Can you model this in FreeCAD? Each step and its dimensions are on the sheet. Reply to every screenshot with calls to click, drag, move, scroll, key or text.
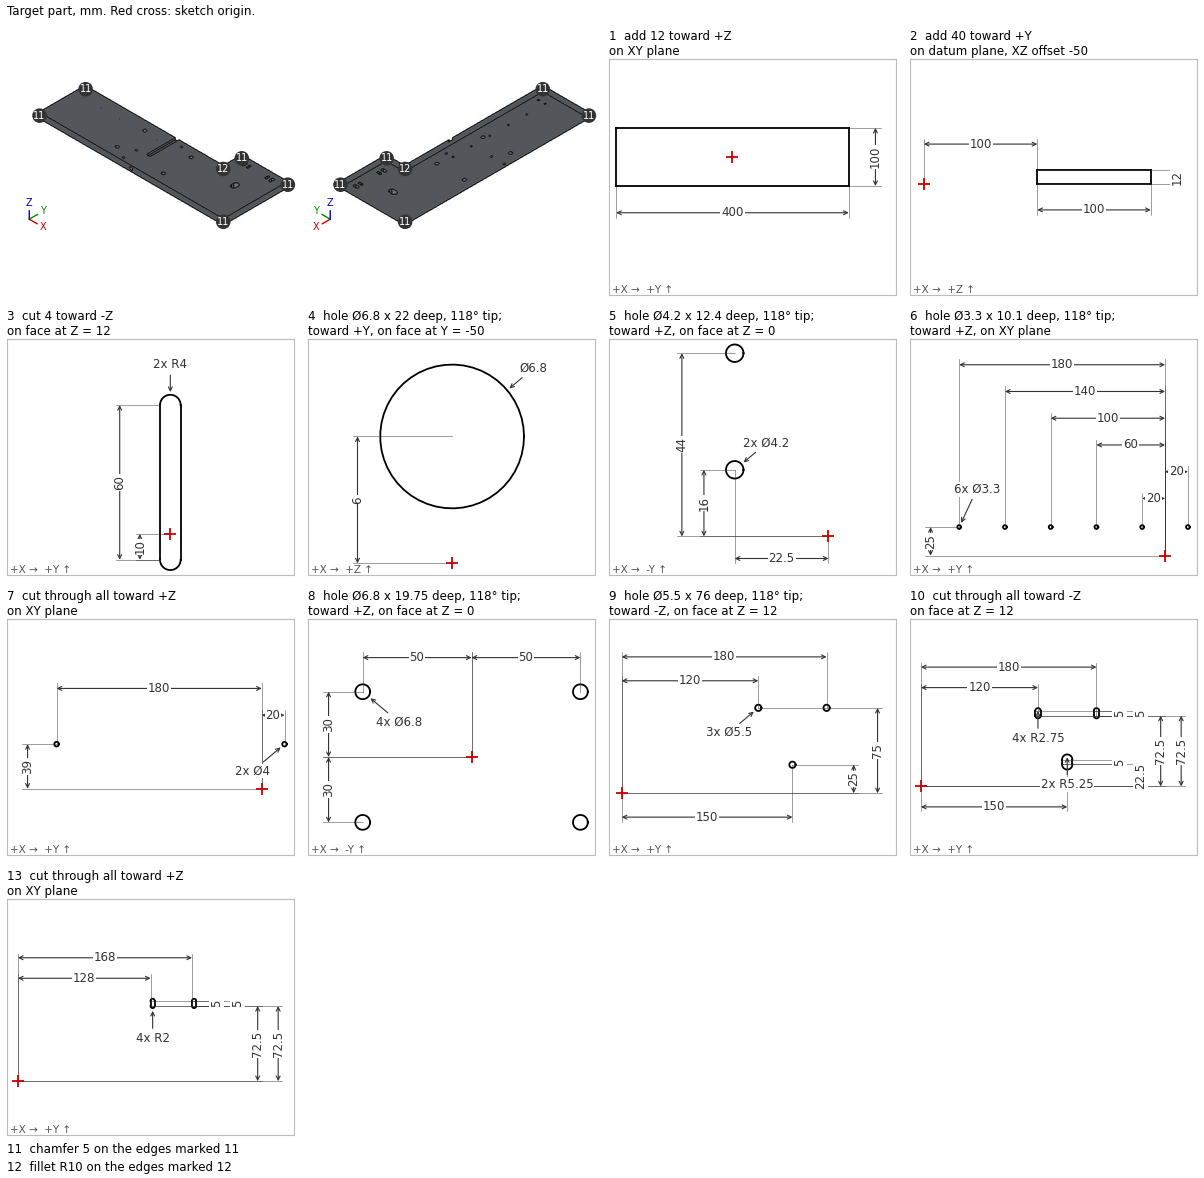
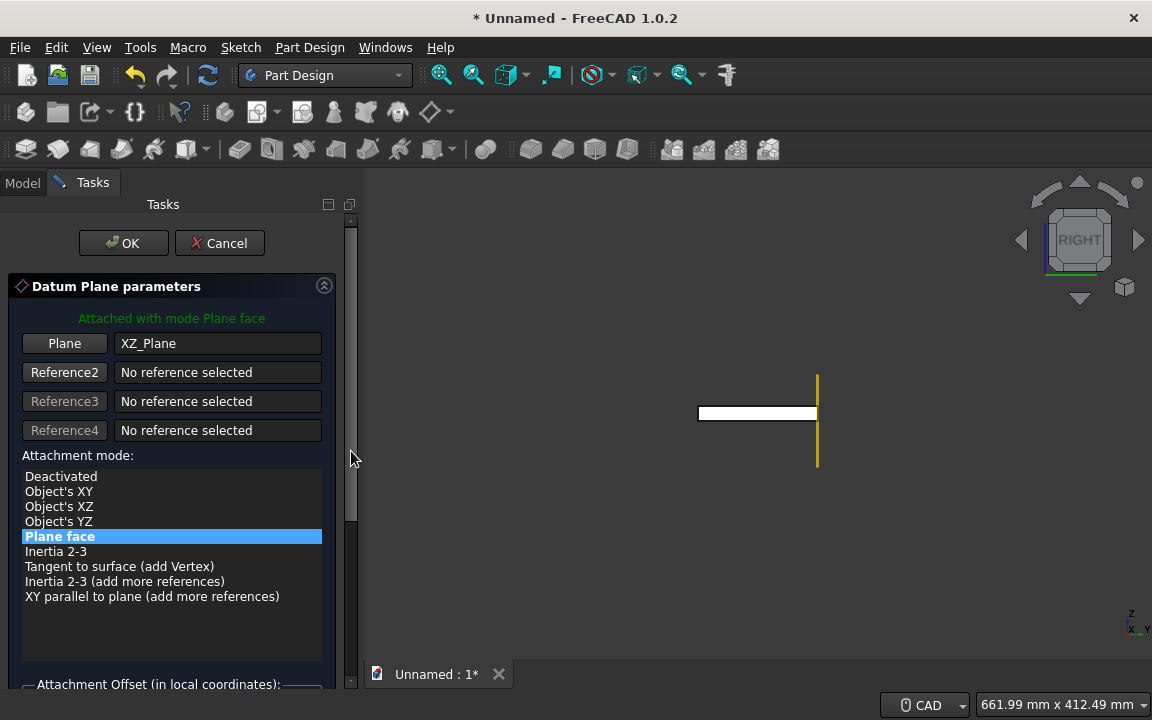
click(124, 243)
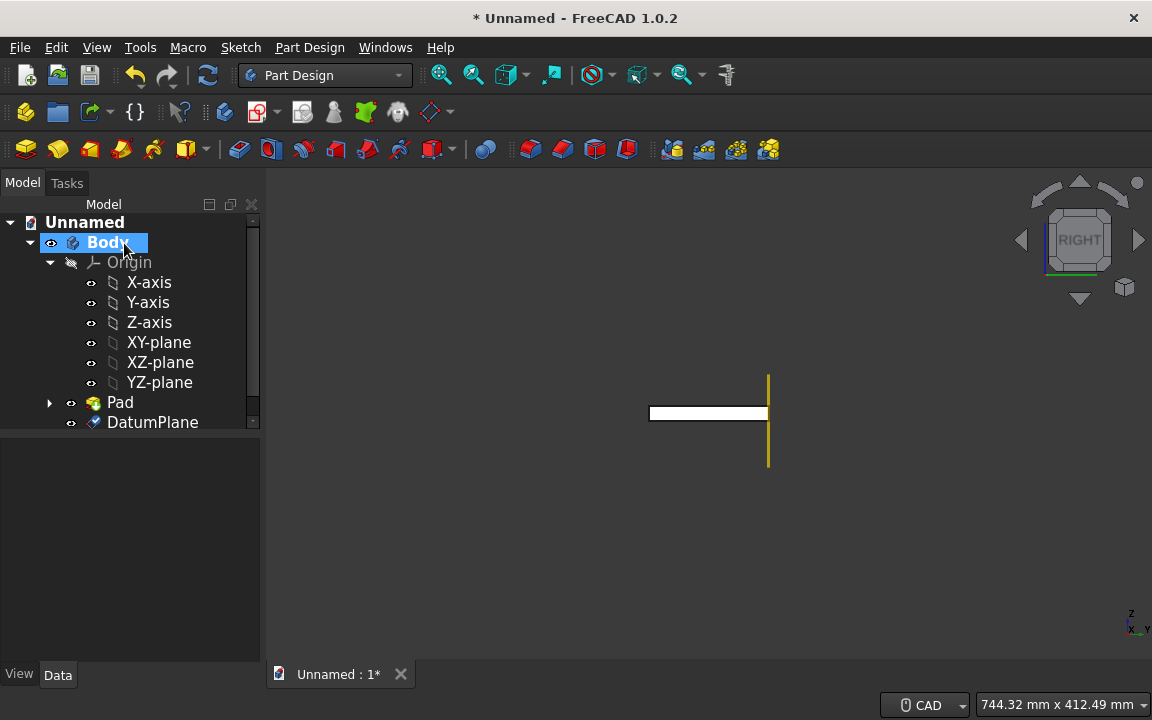
click(116, 423)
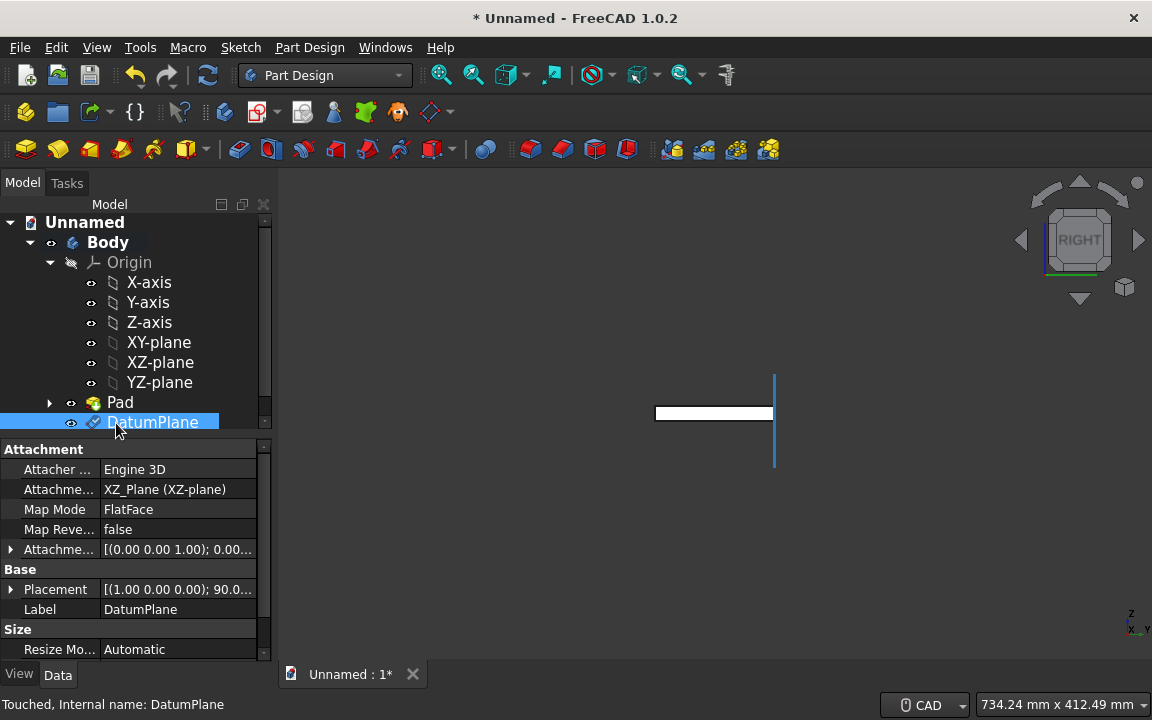
click(258, 112)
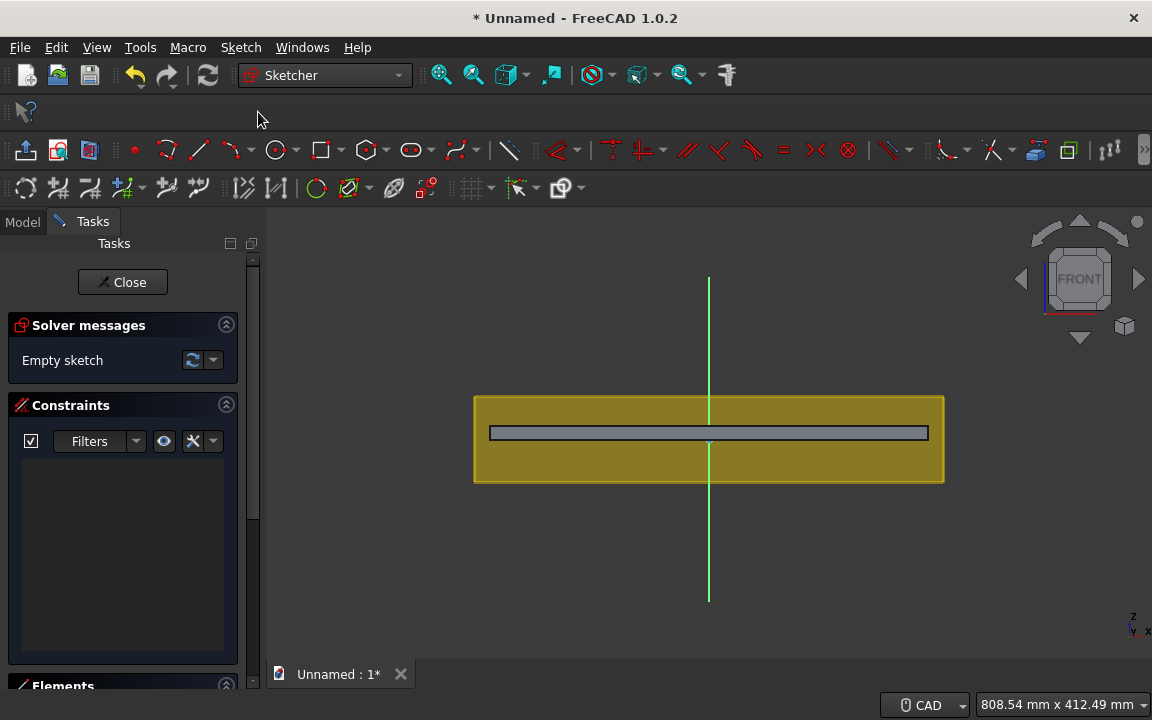
click(90, 150)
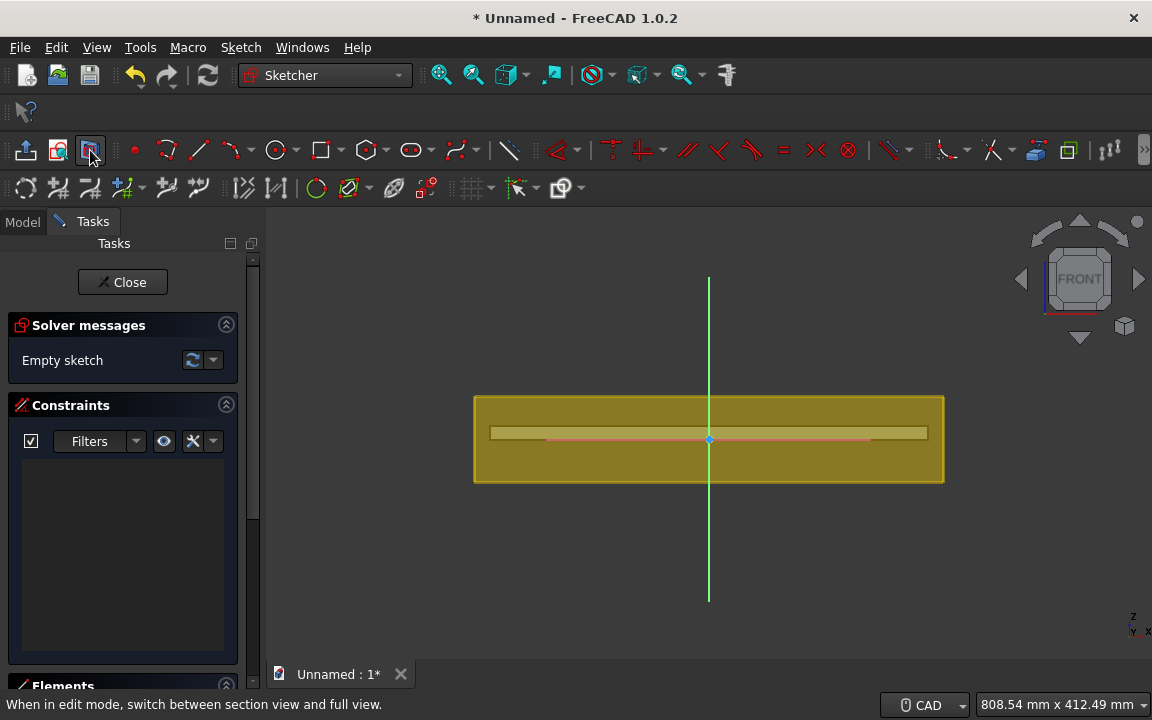
scroll(964, 433, up, 4)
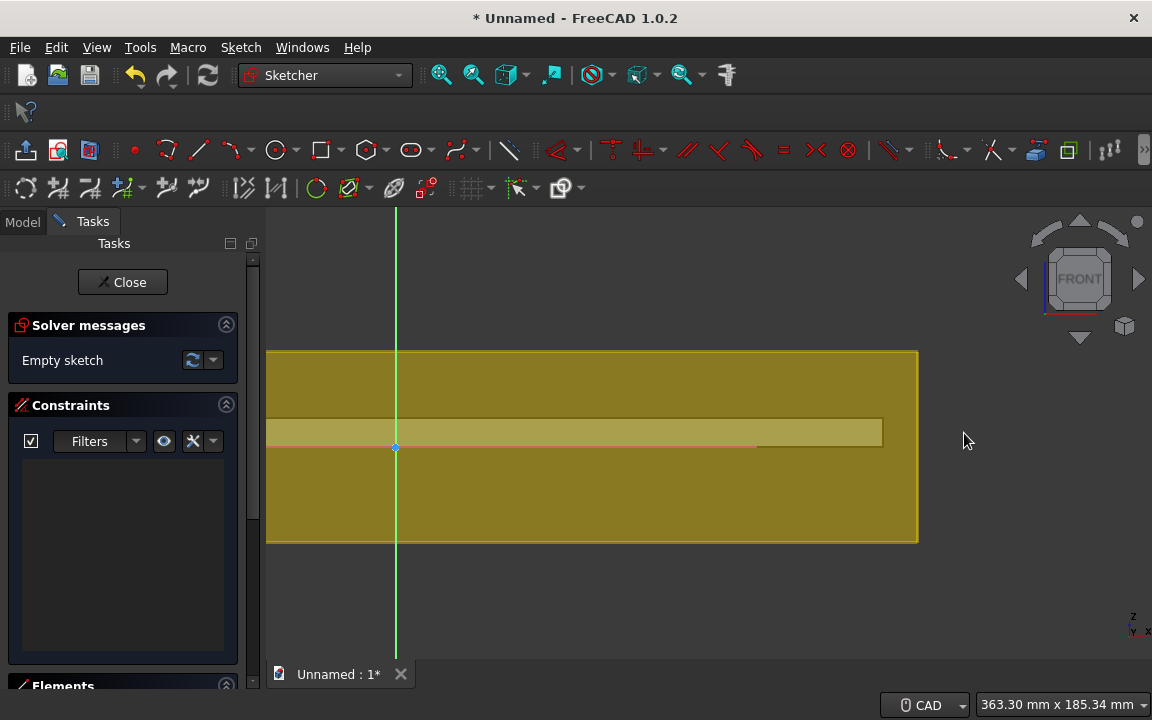
click(322, 150)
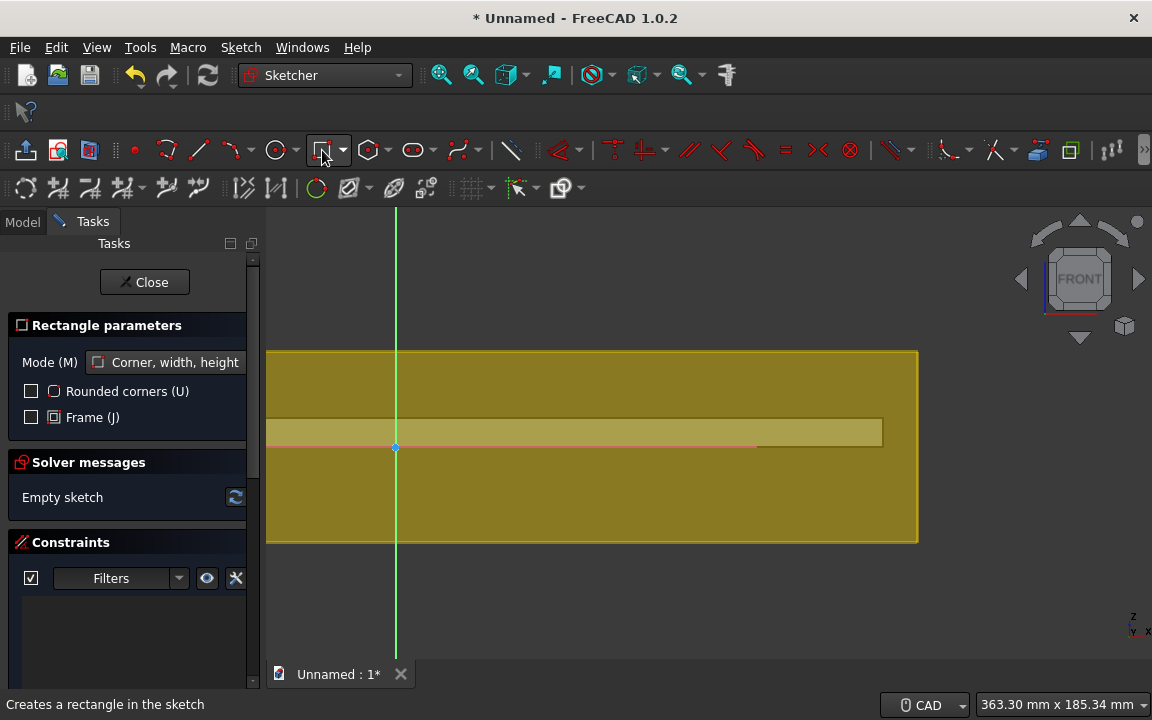
click(639, 418)
click(883, 447)
key(Escape)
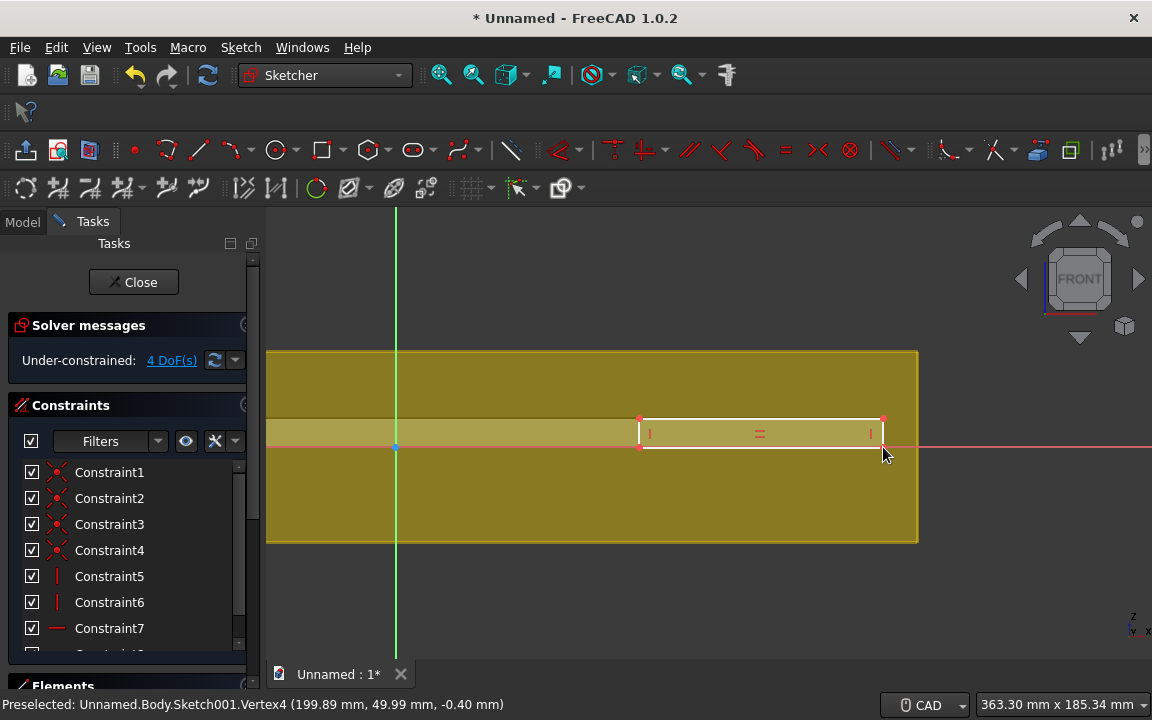
click(639, 448)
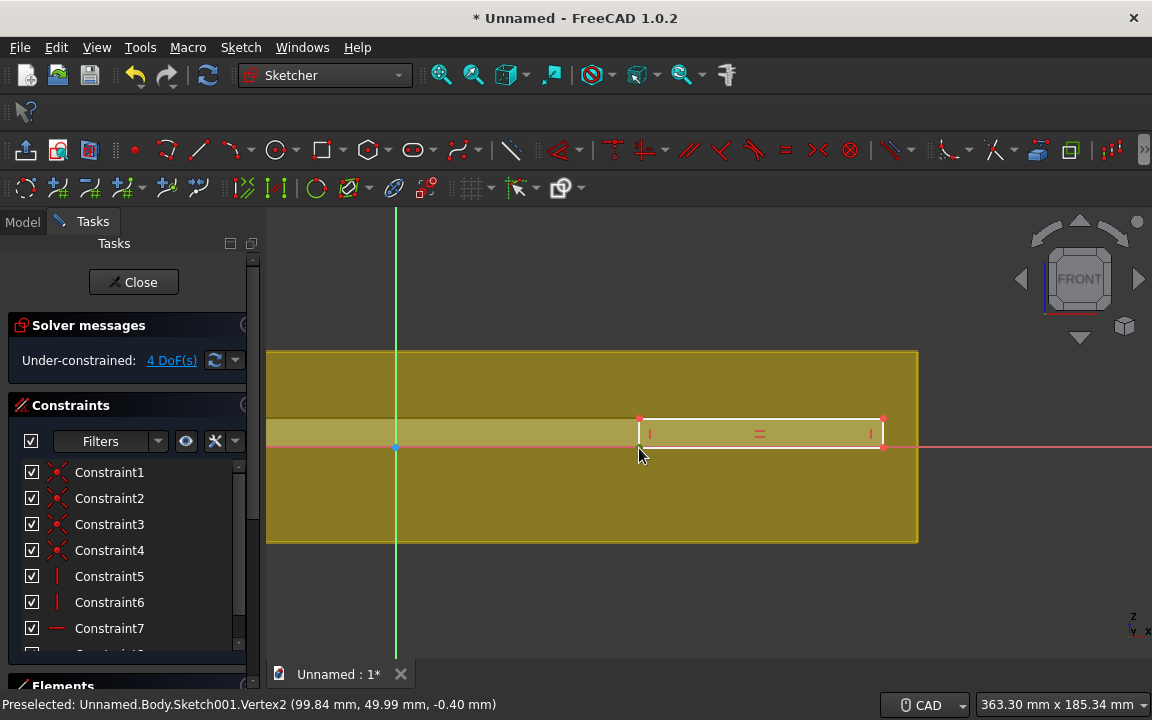
click(344, 447)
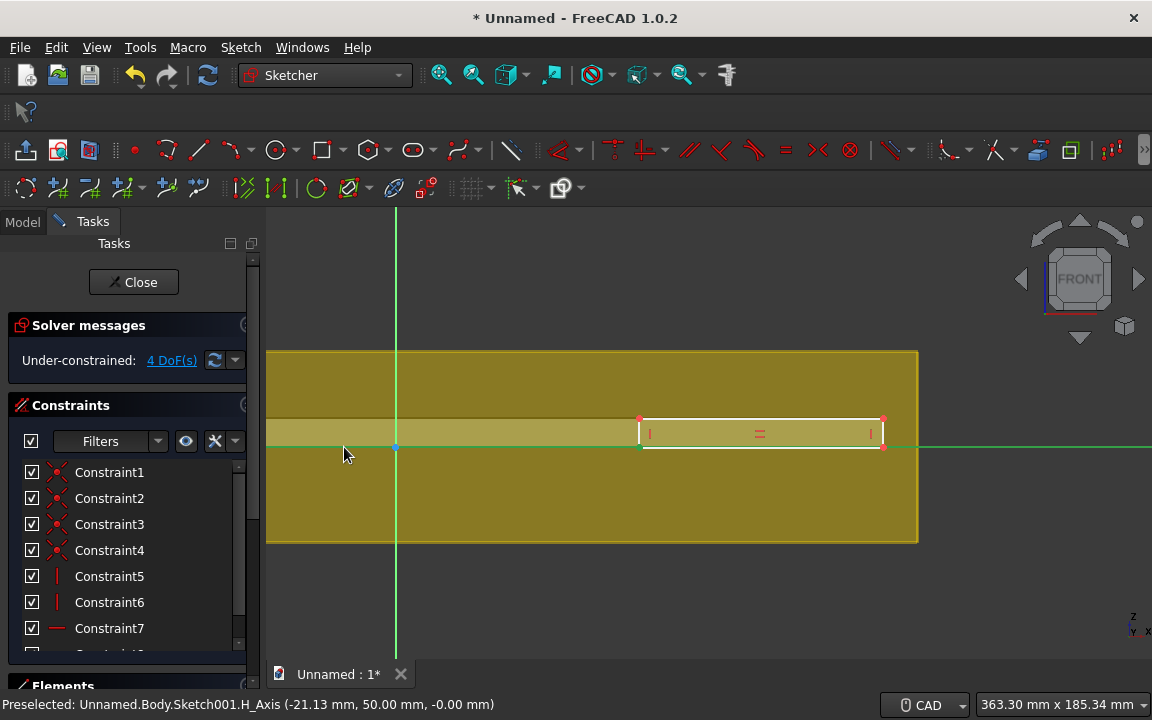
click(614, 150)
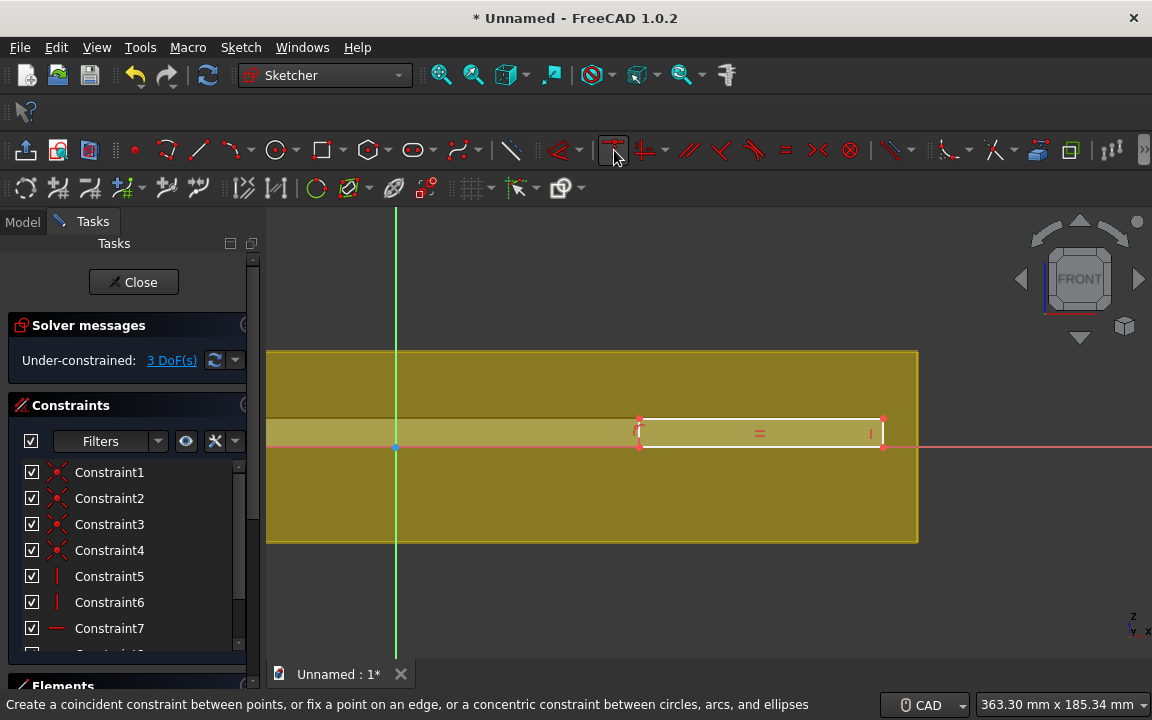
click(558, 150)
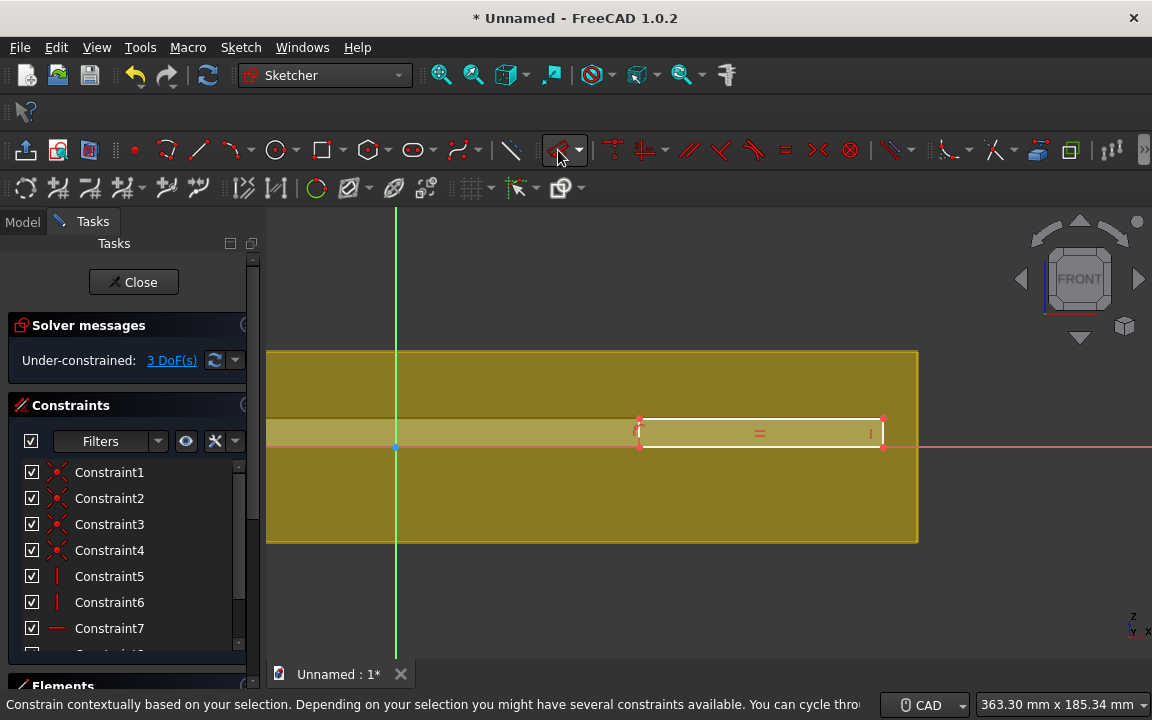
scroll(639, 430, up, 2)